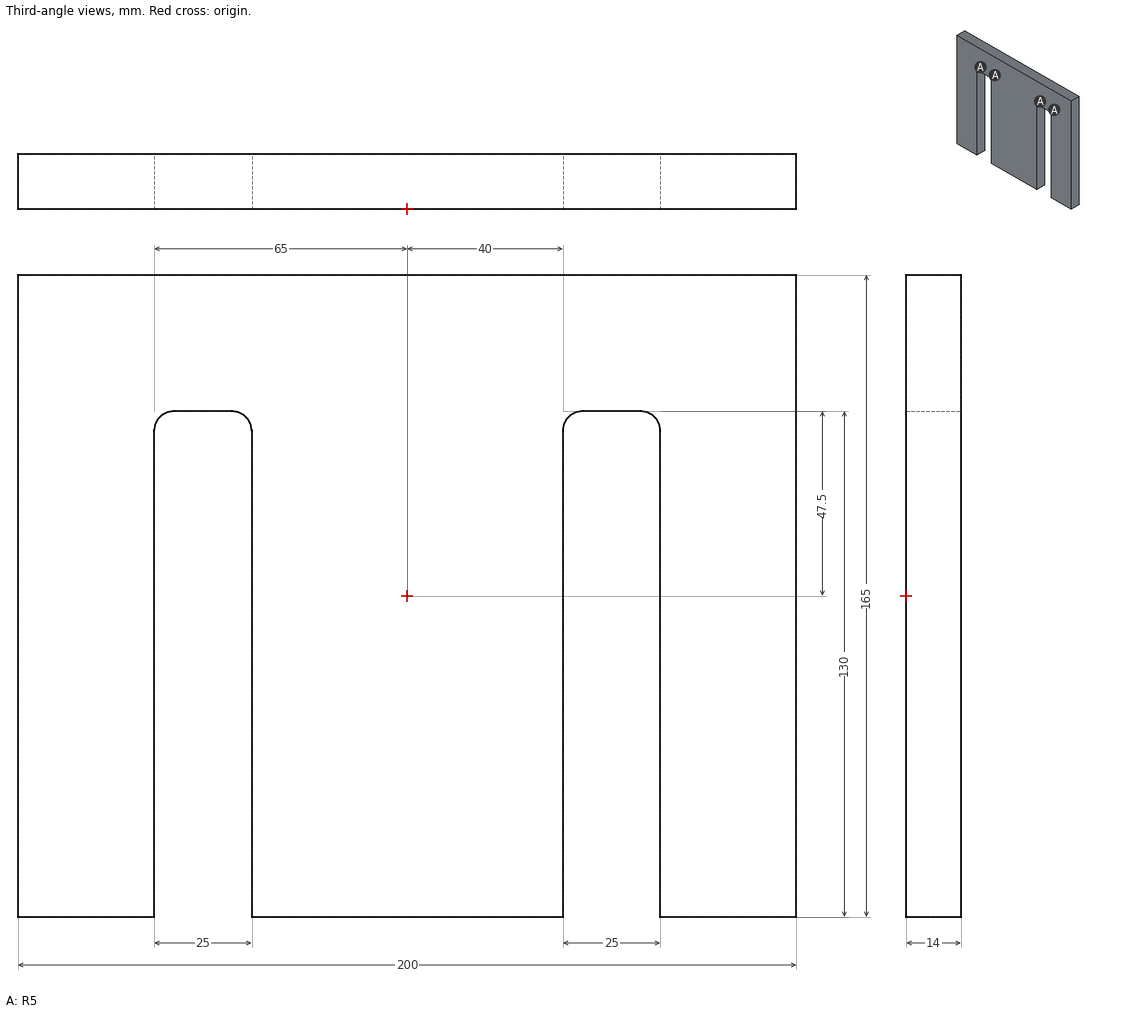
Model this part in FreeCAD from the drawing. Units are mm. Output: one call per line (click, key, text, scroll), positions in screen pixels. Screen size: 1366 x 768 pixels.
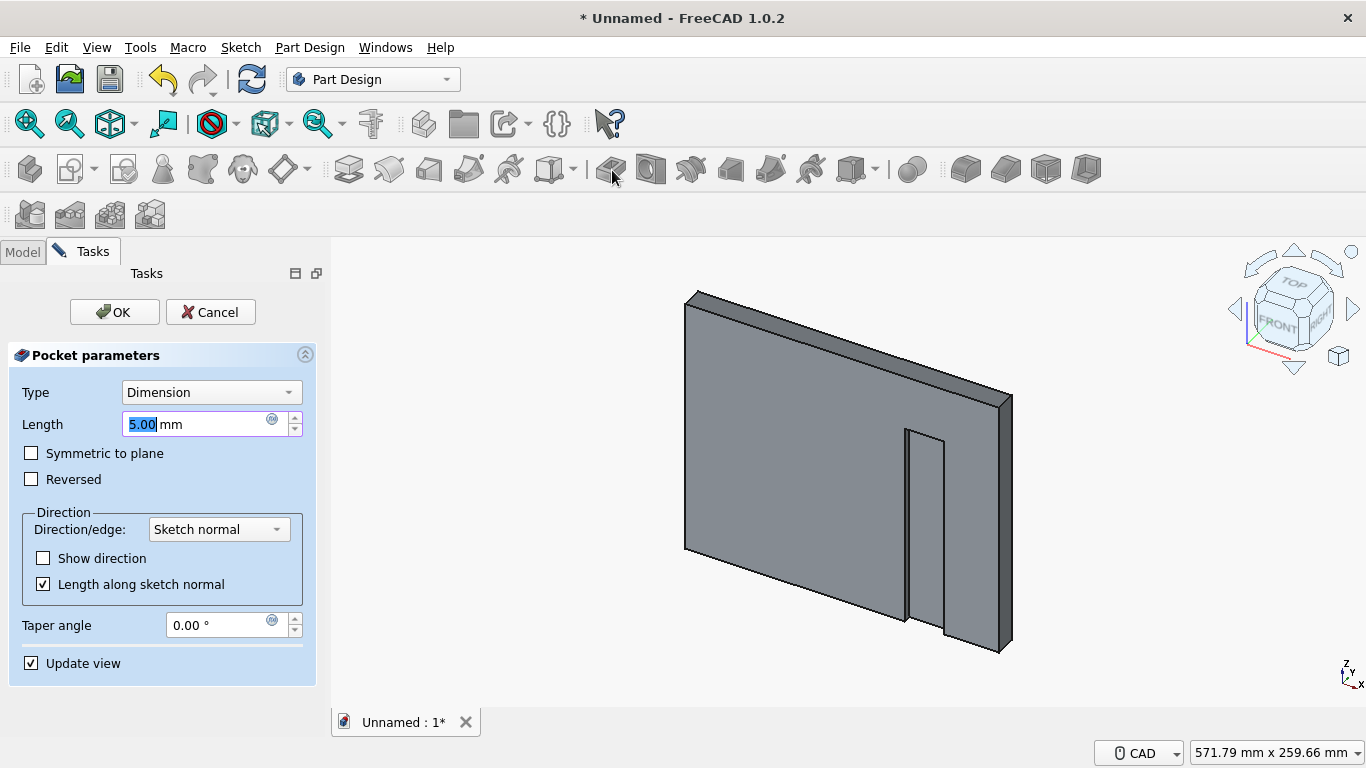
click(212, 392)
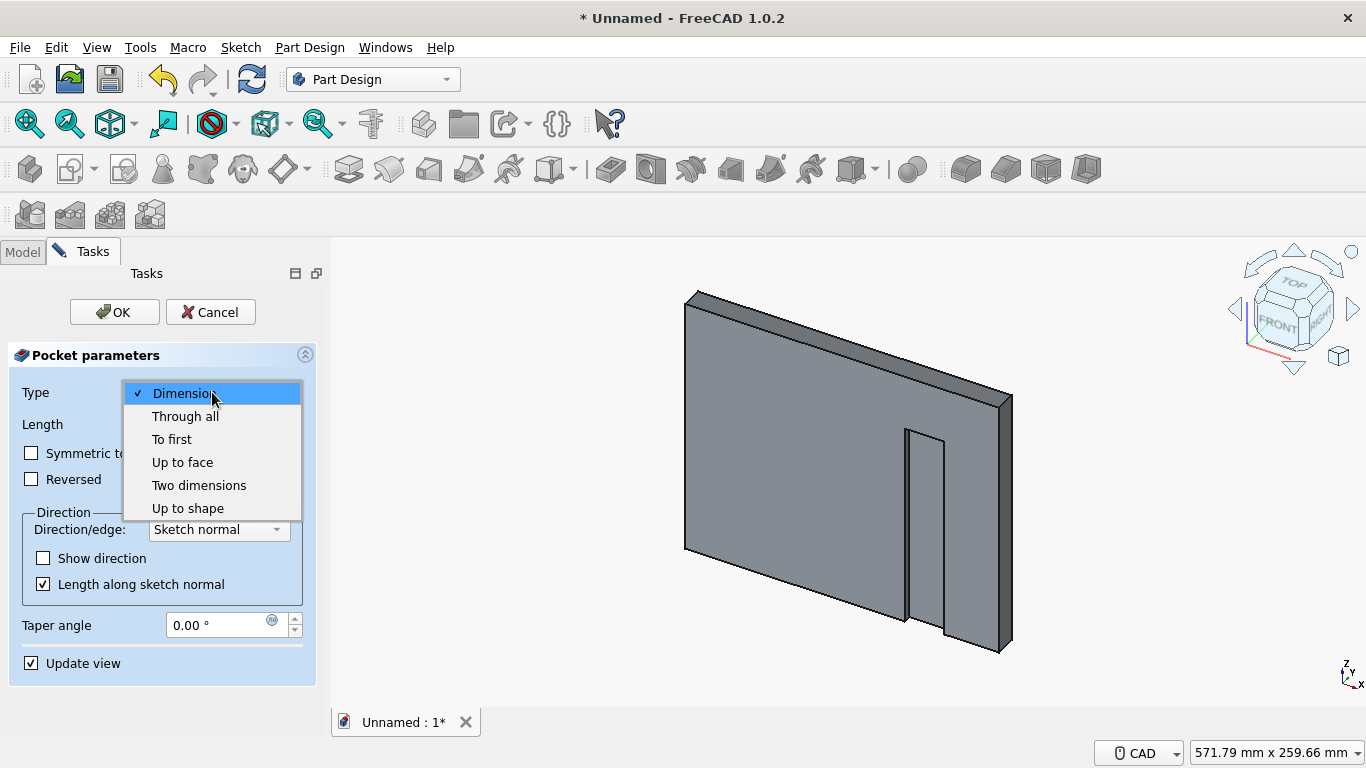
click(212, 440)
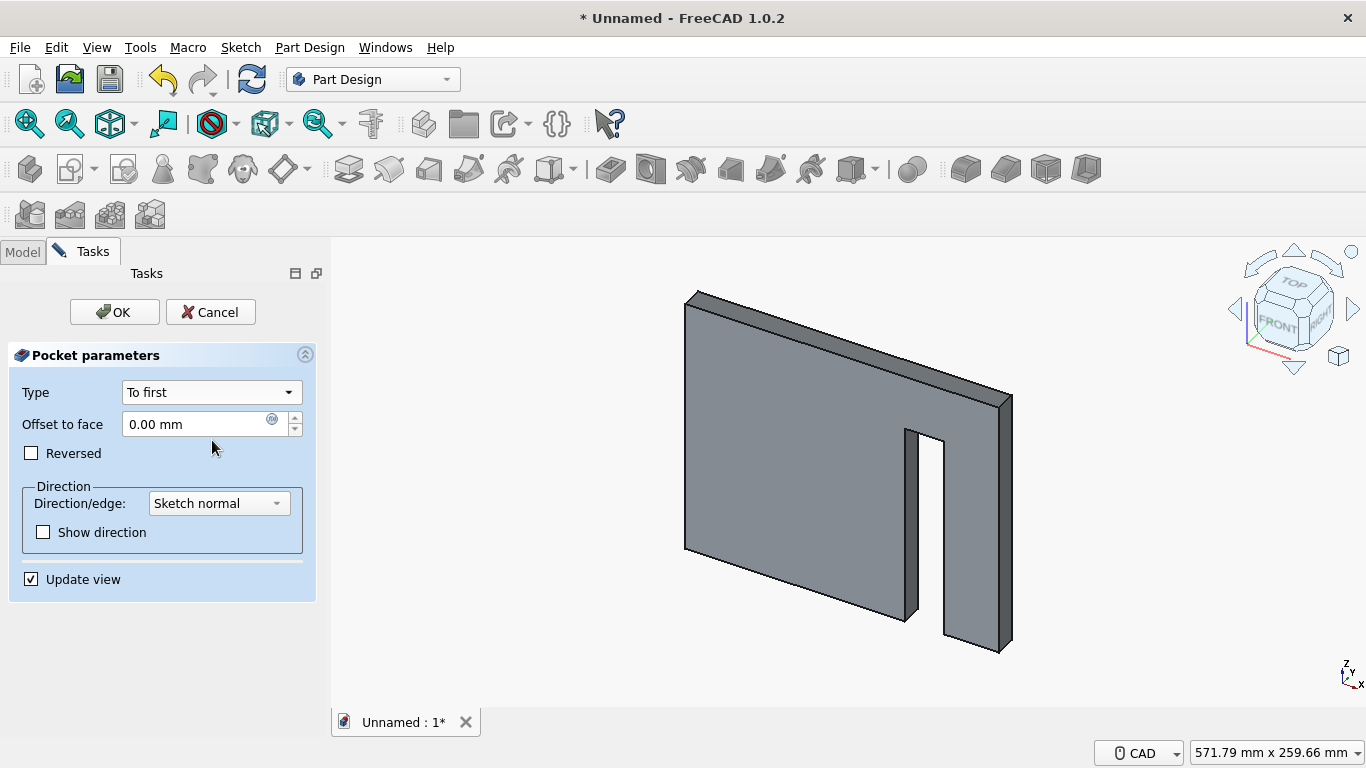
click(115, 312)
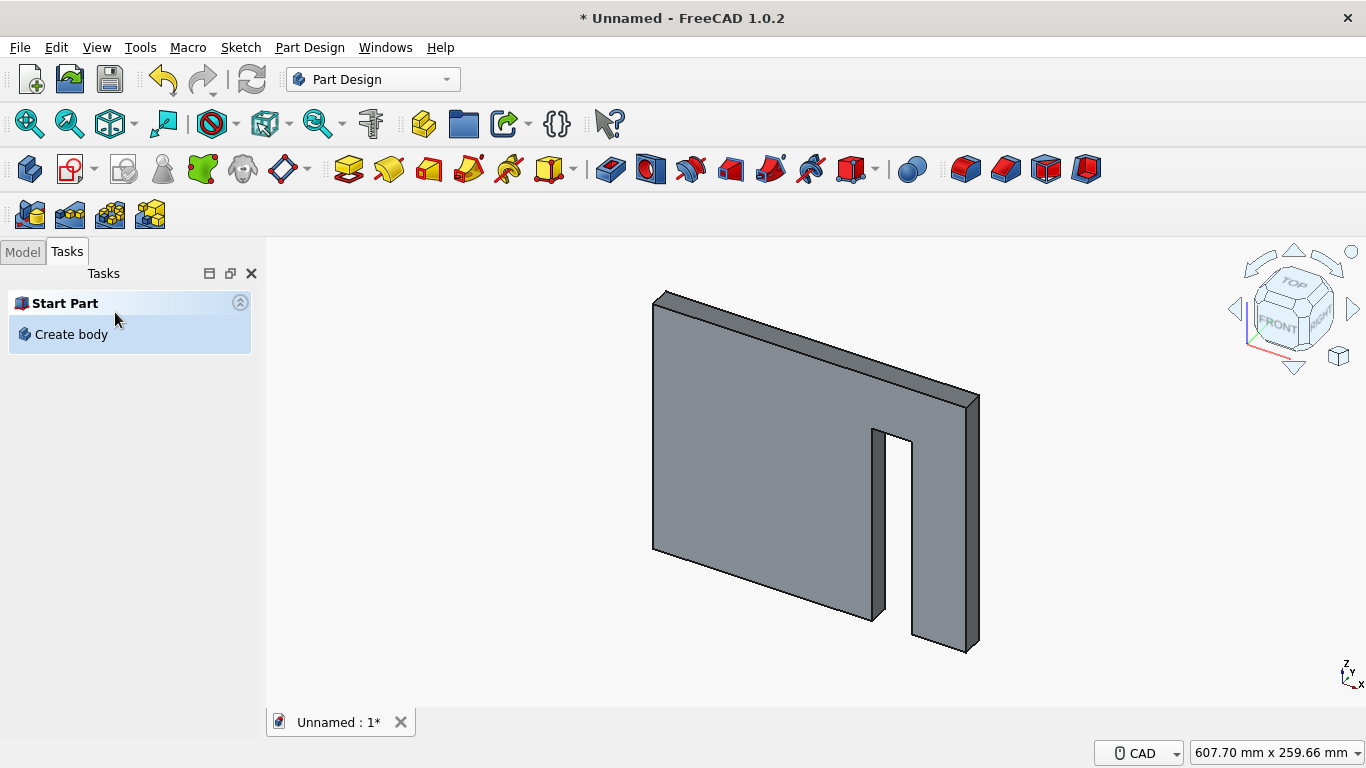
click(70, 170)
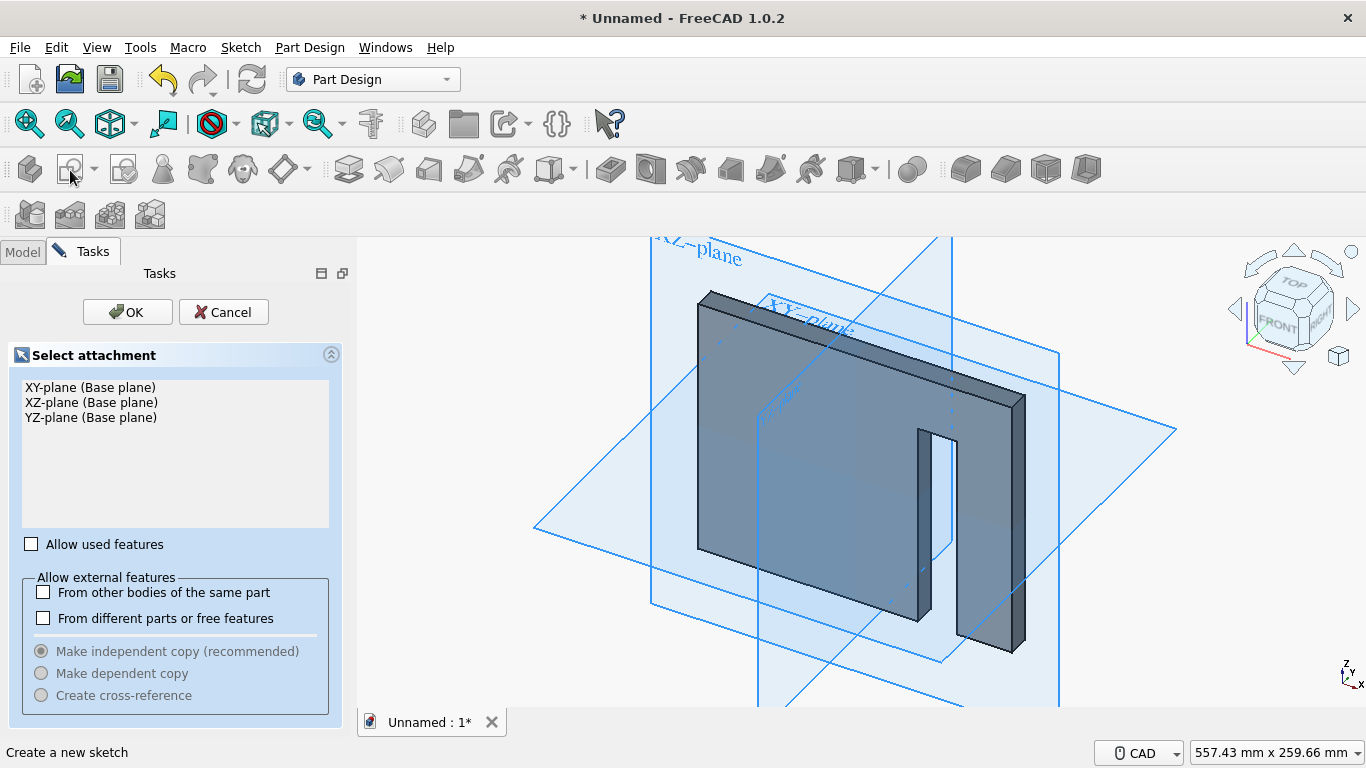
click(82, 402)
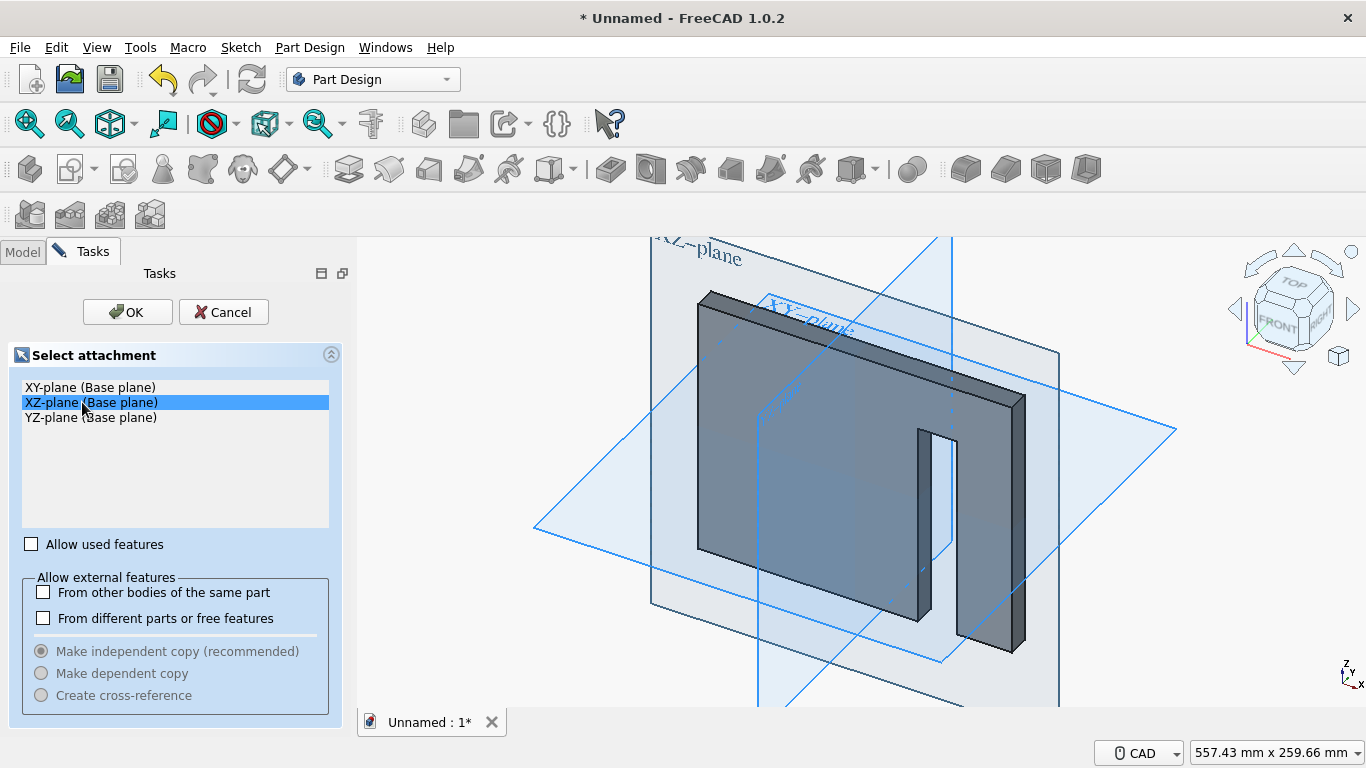
click(128, 312)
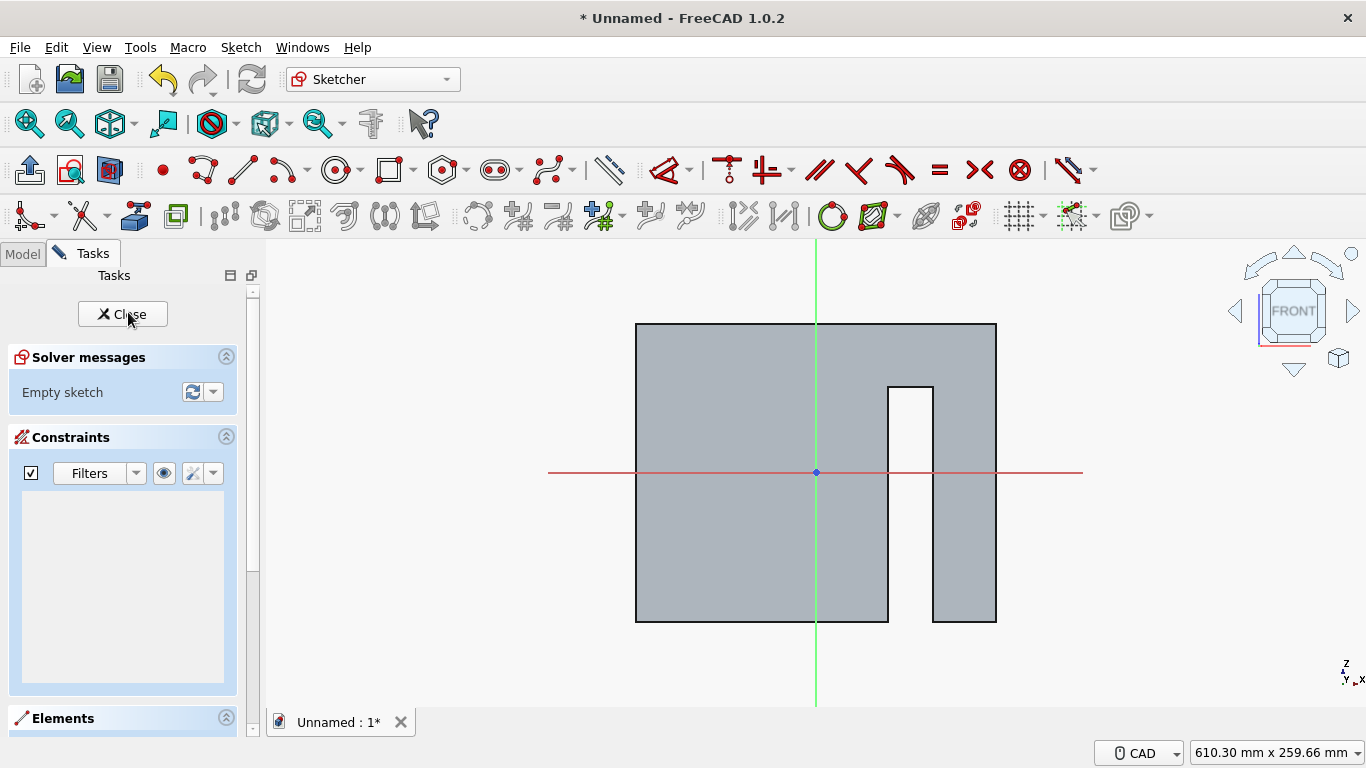
click(390, 170)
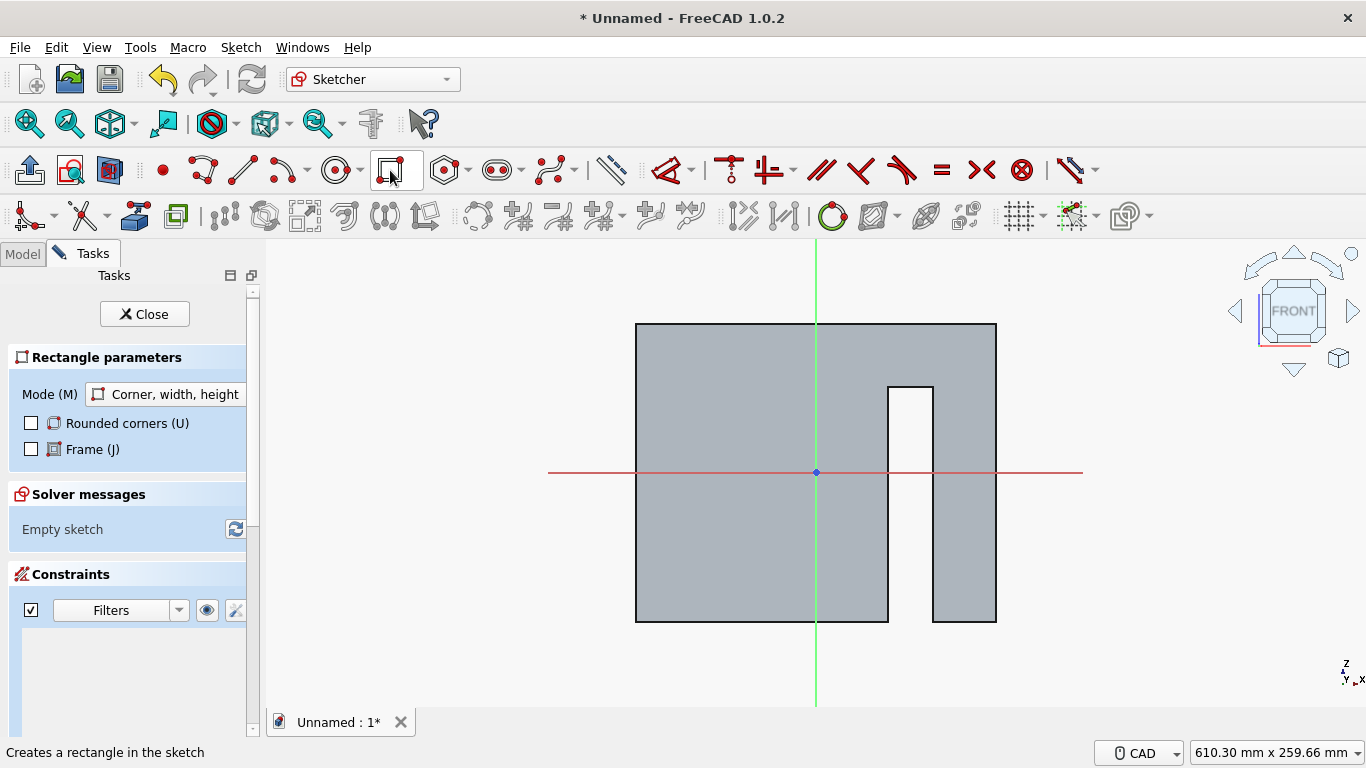
click(699, 387)
move(744, 622)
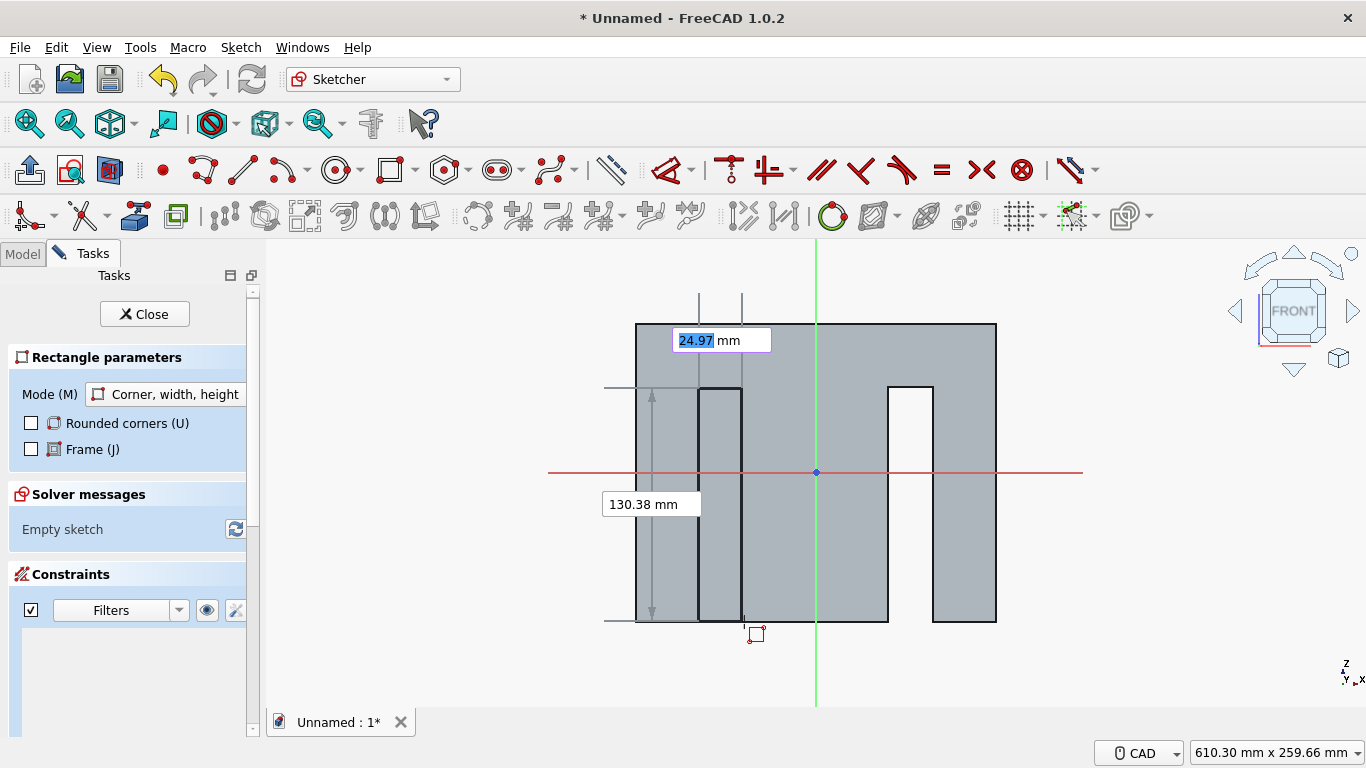
text(25)
key(Tab)
text(130)
key(Return)
key(Escape)